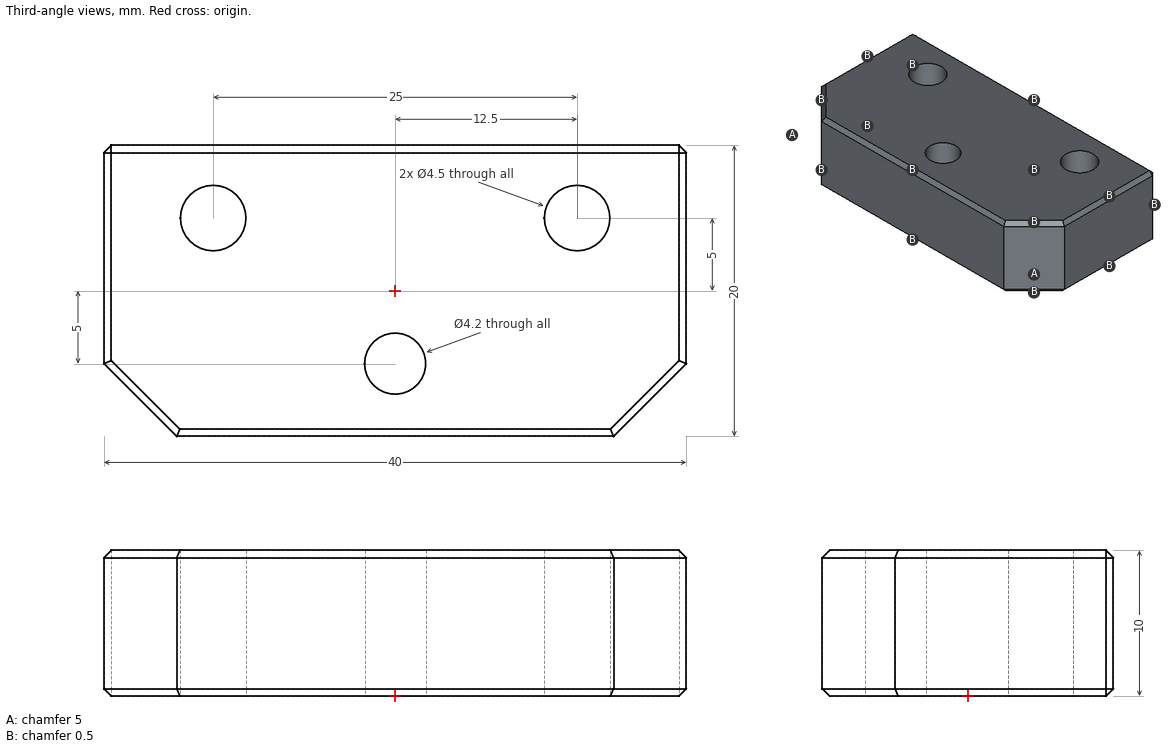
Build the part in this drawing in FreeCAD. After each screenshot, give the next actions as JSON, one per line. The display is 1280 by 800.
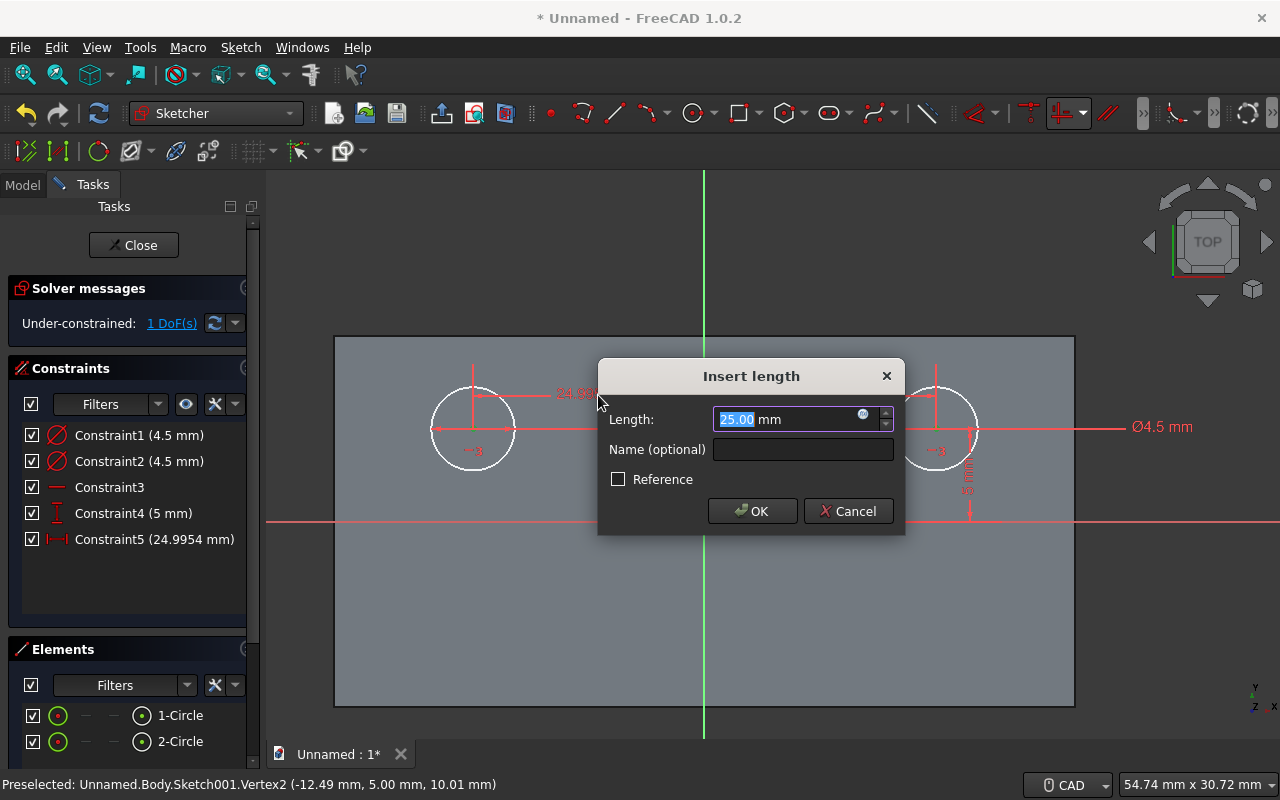
{"action": "type", "text": "25"}
{"action": "key", "text": "Return"}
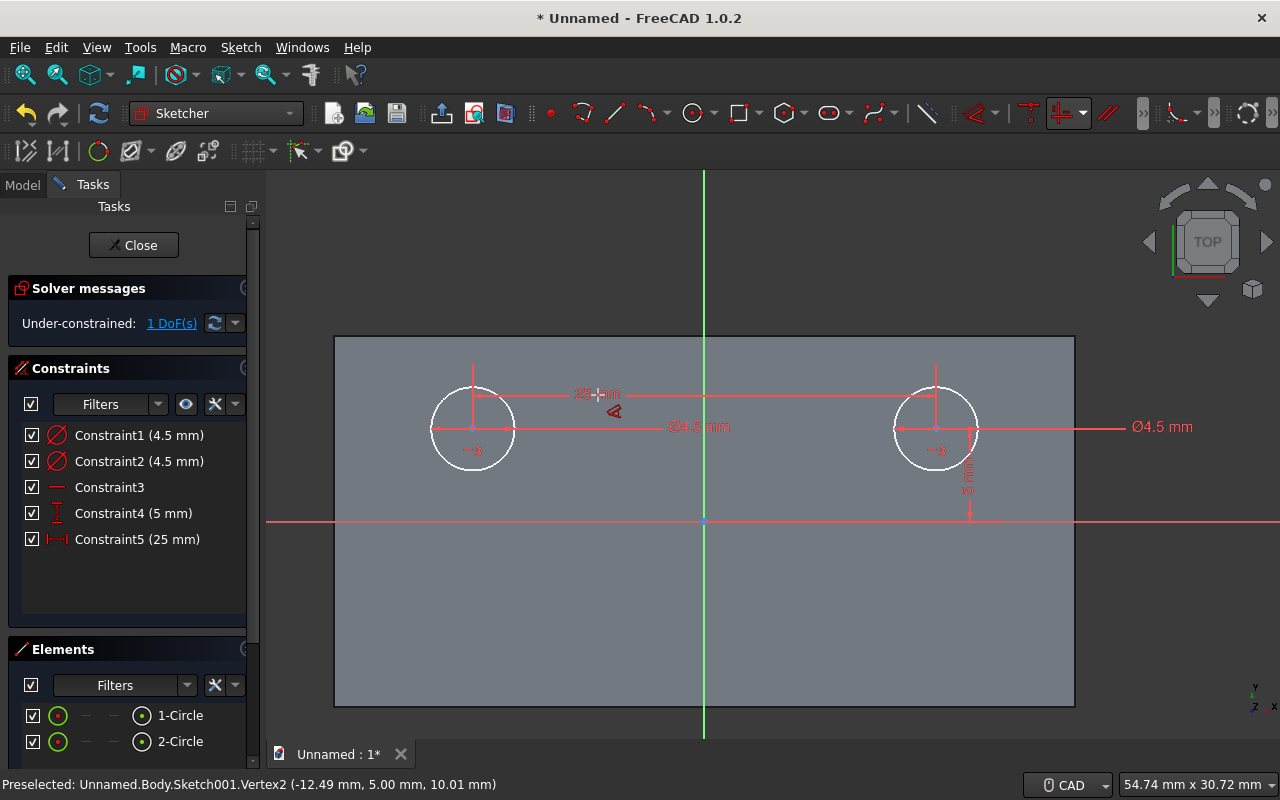
{"action": "left_click", "coordinate": [936, 429]}
{"action": "left_click", "coordinate": [820, 556]}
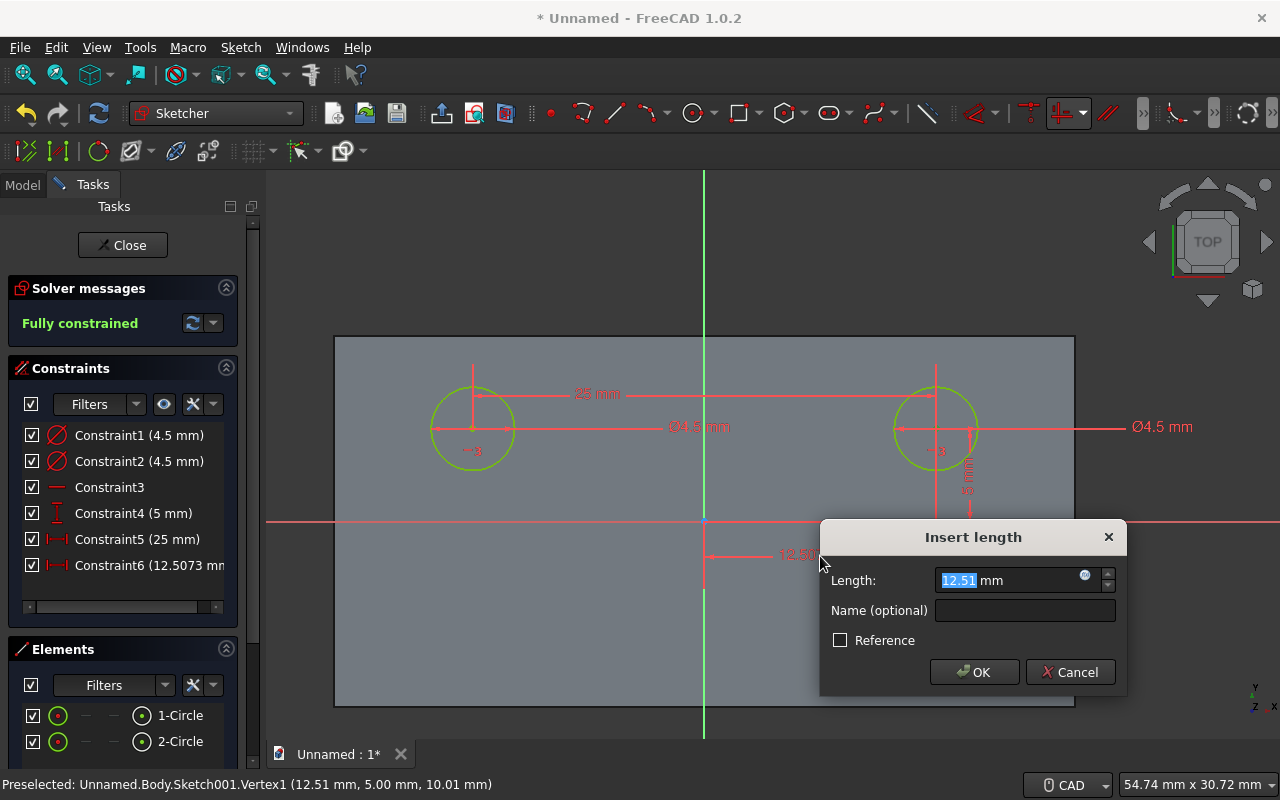
{"action": "type", "text": "12.5"}
{"action": "key", "text": "Return"}
{"action": "key", "text": "Escape"}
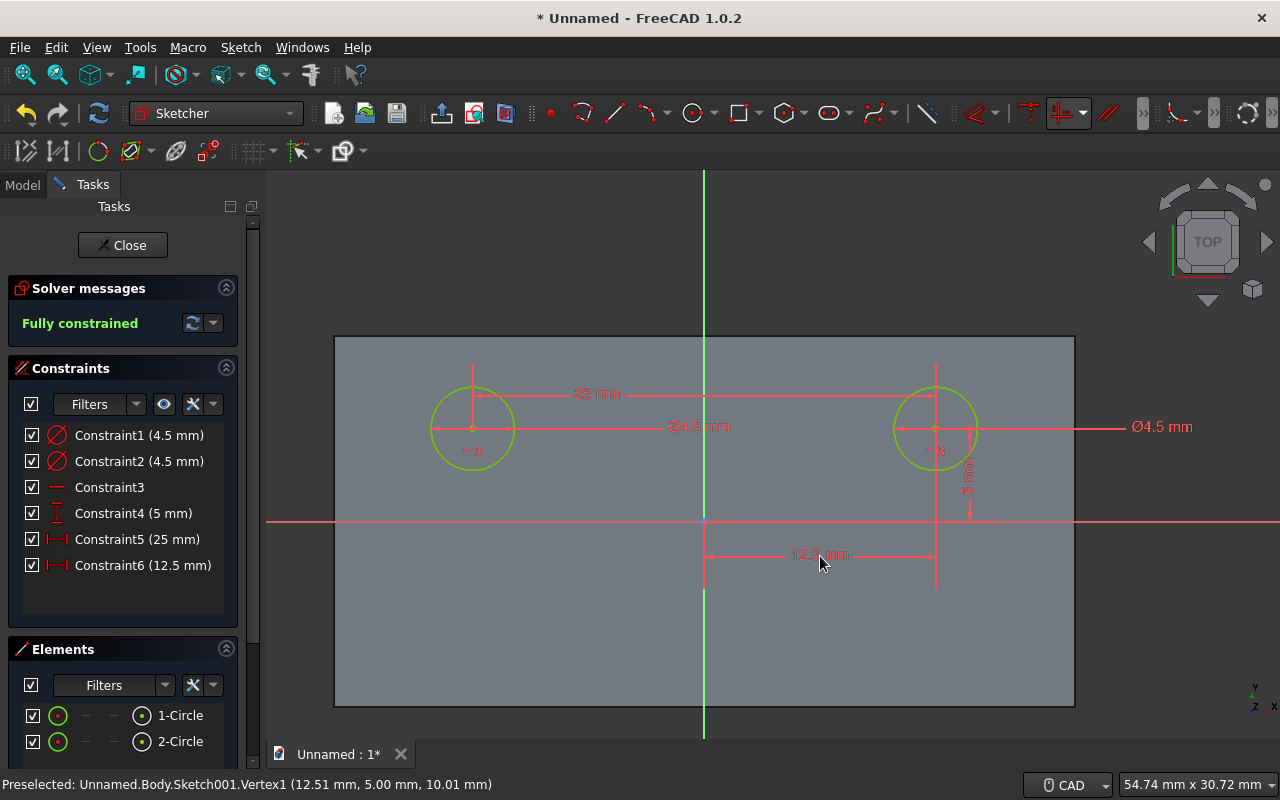
{"action": "left_click", "coordinate": [123, 245]}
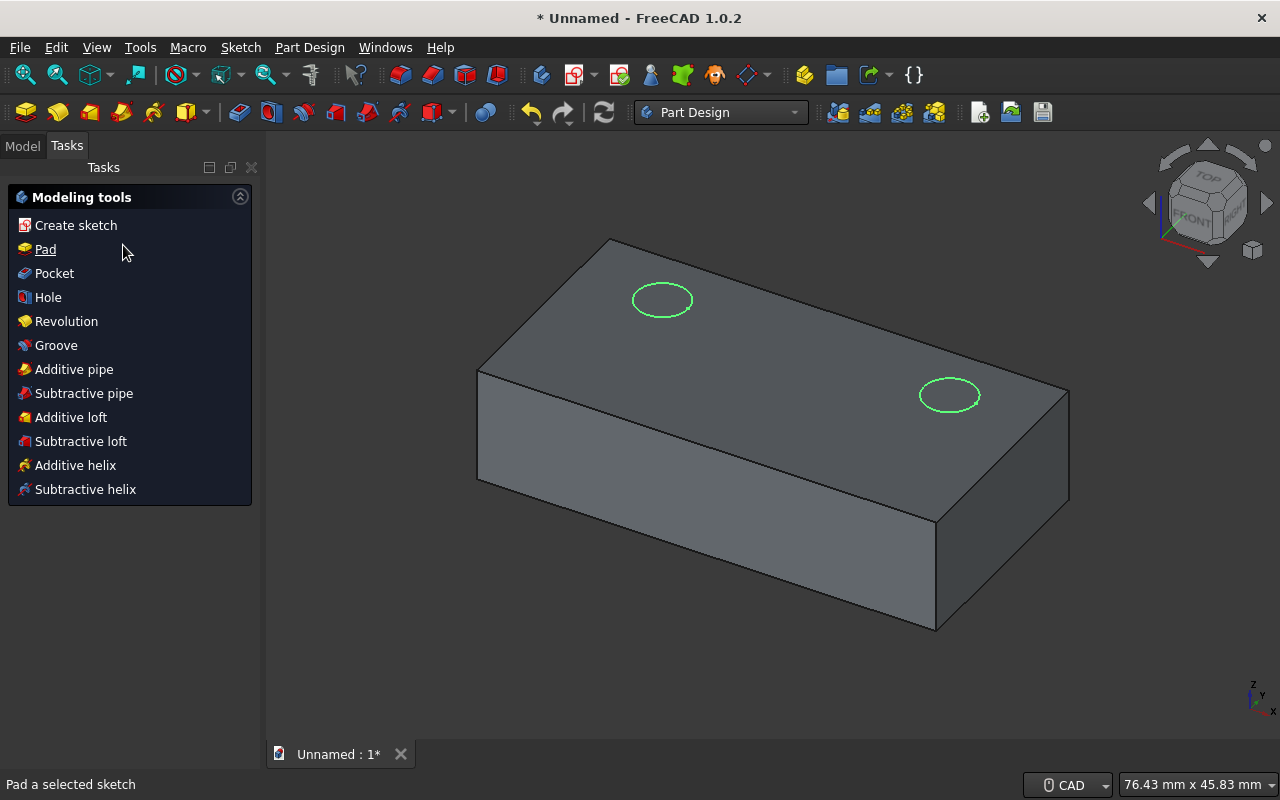
{"action": "left_click", "coordinate": [272, 112]}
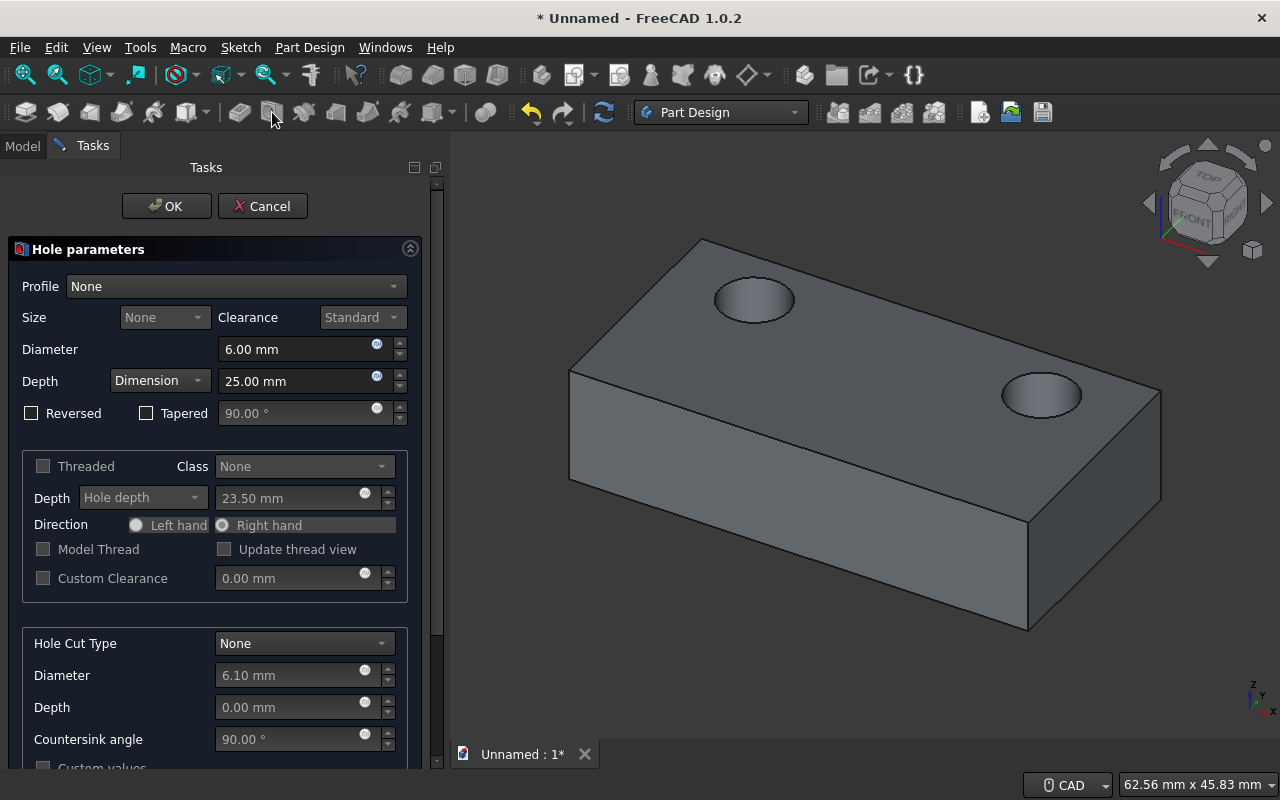
{"action": "triple_click", "coordinate": [305, 349]}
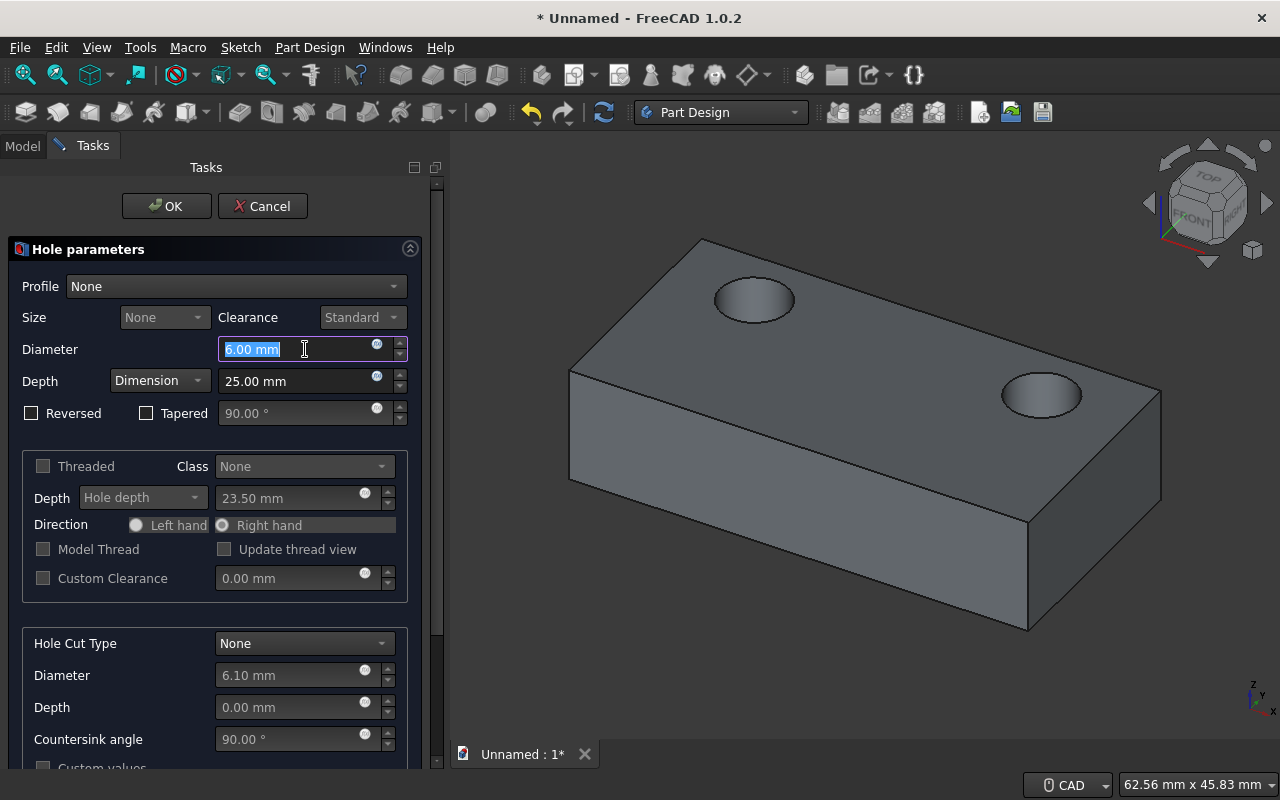
{"action": "type", "text": "4.5"}
{"action": "key", "text": "Tab"}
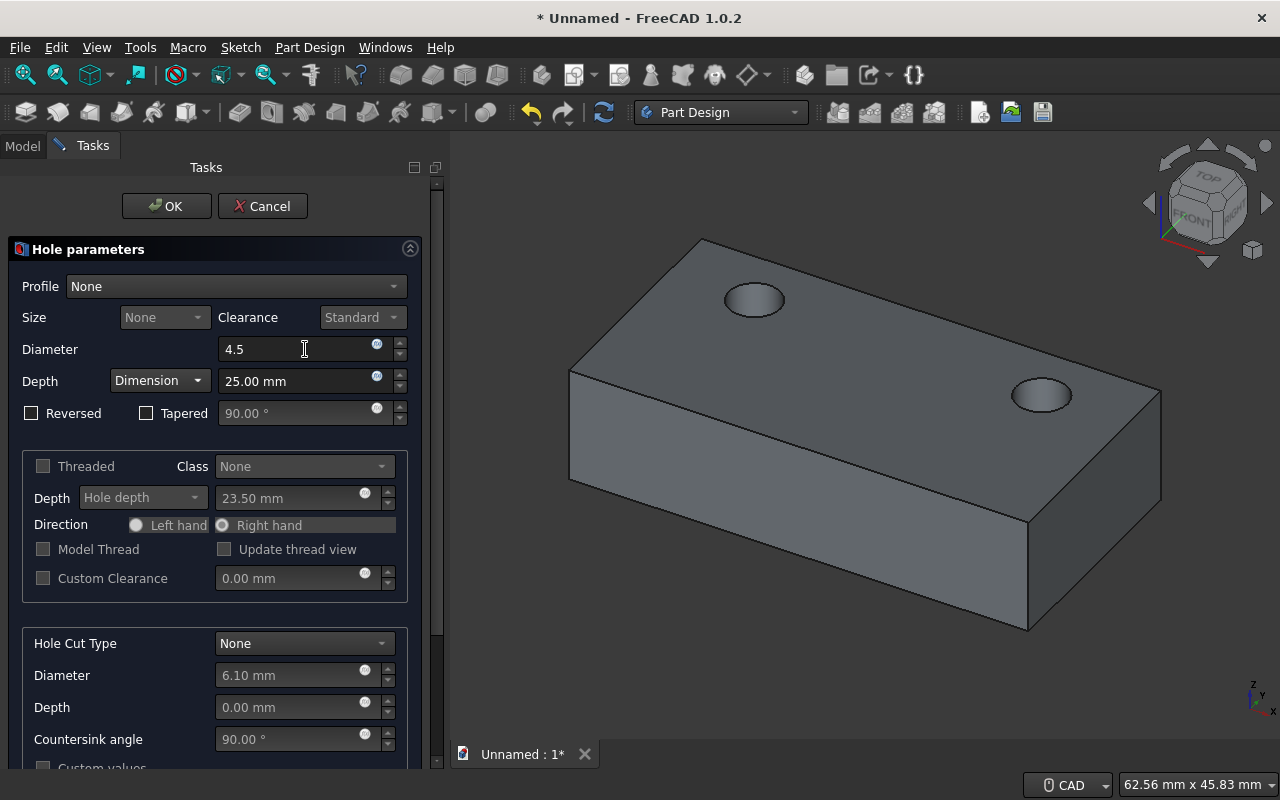
{"action": "left_click", "coordinate": [161, 380]}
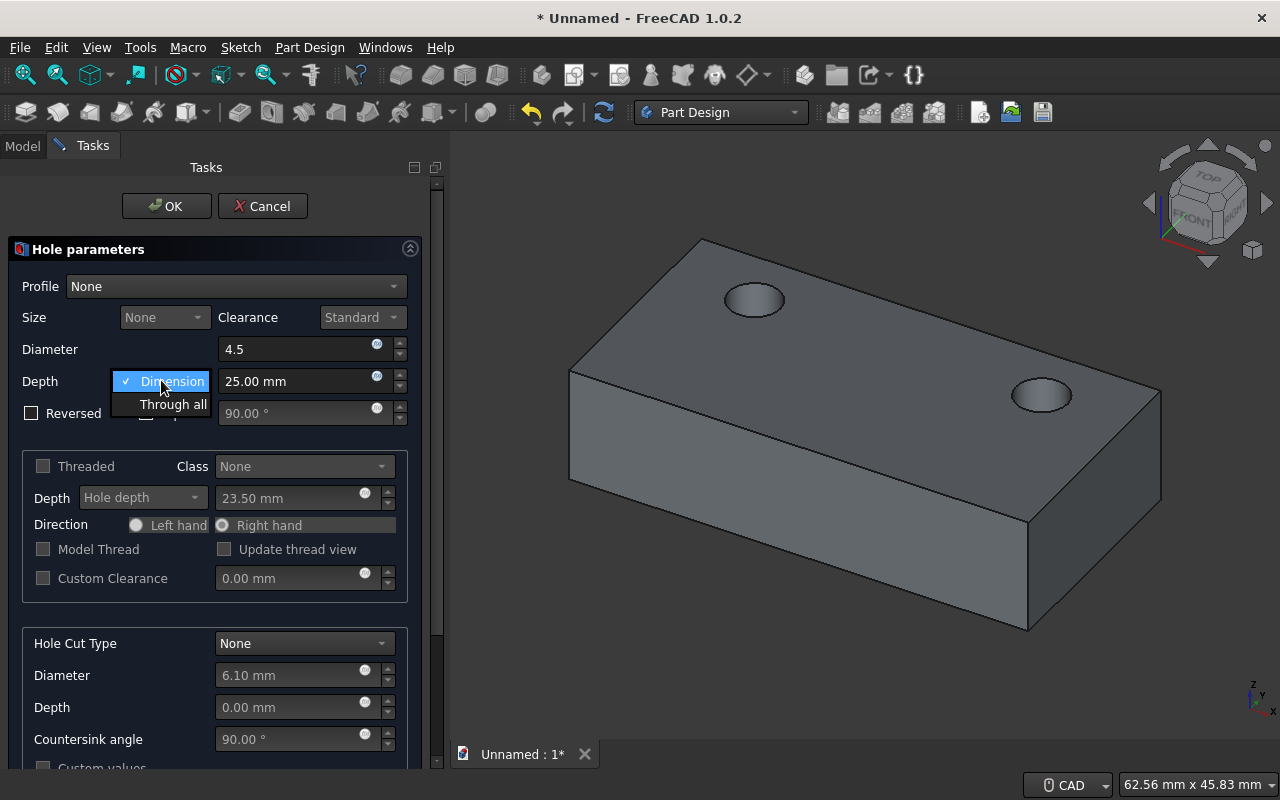
{"action": "left_click", "coordinate": [160, 404]}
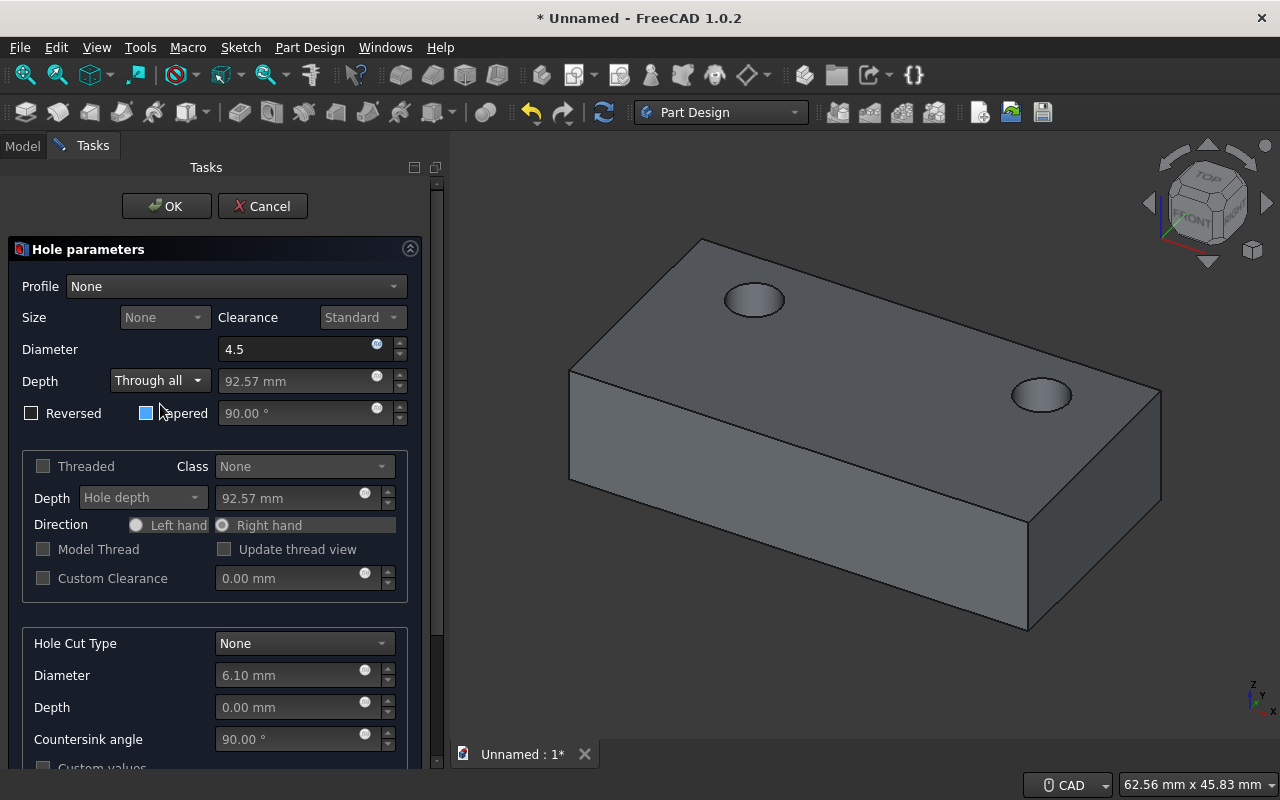
{"action": "left_click", "coordinate": [167, 206]}